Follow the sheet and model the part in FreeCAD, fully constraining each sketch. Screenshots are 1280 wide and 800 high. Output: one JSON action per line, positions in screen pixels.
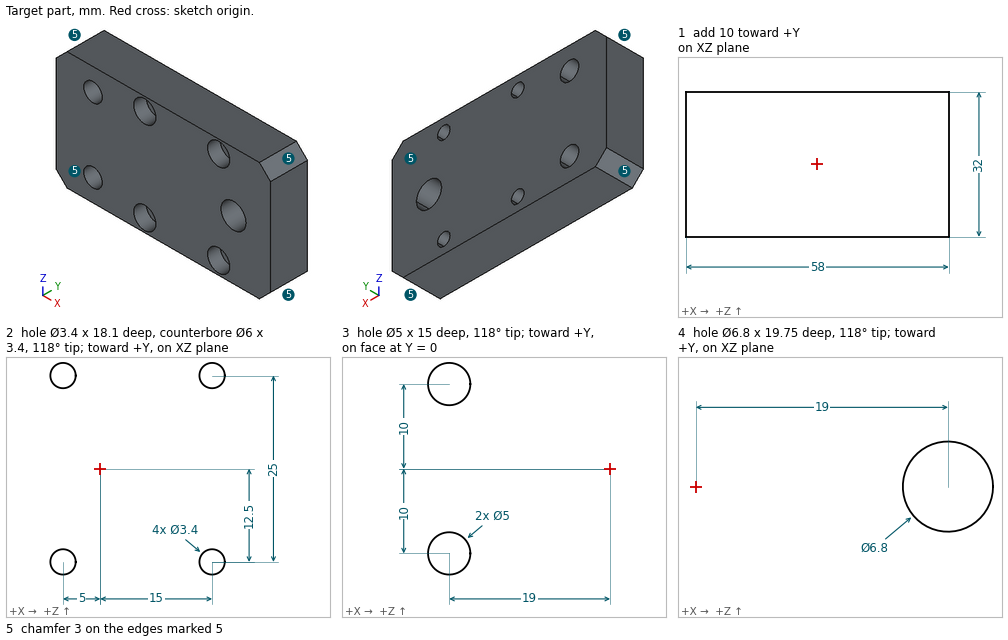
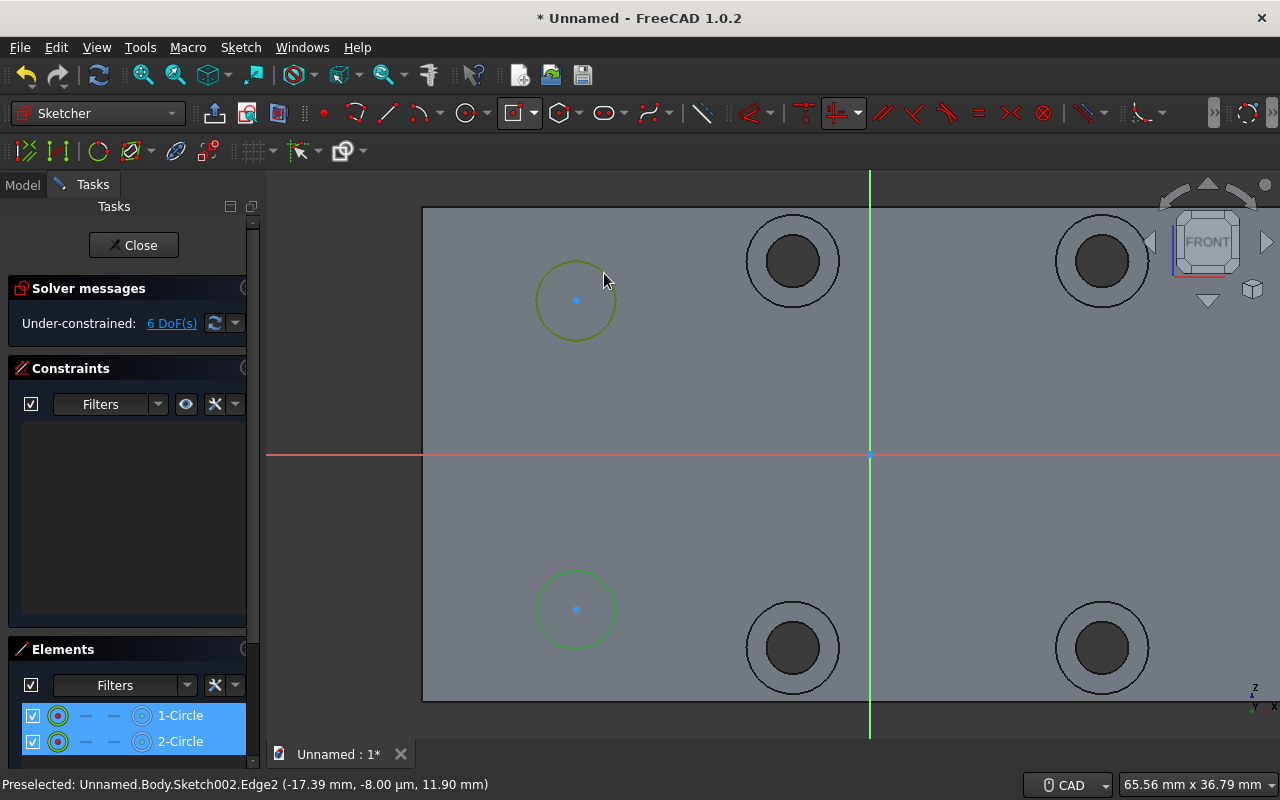
{"action": "left_click", "coordinate": [980, 114]}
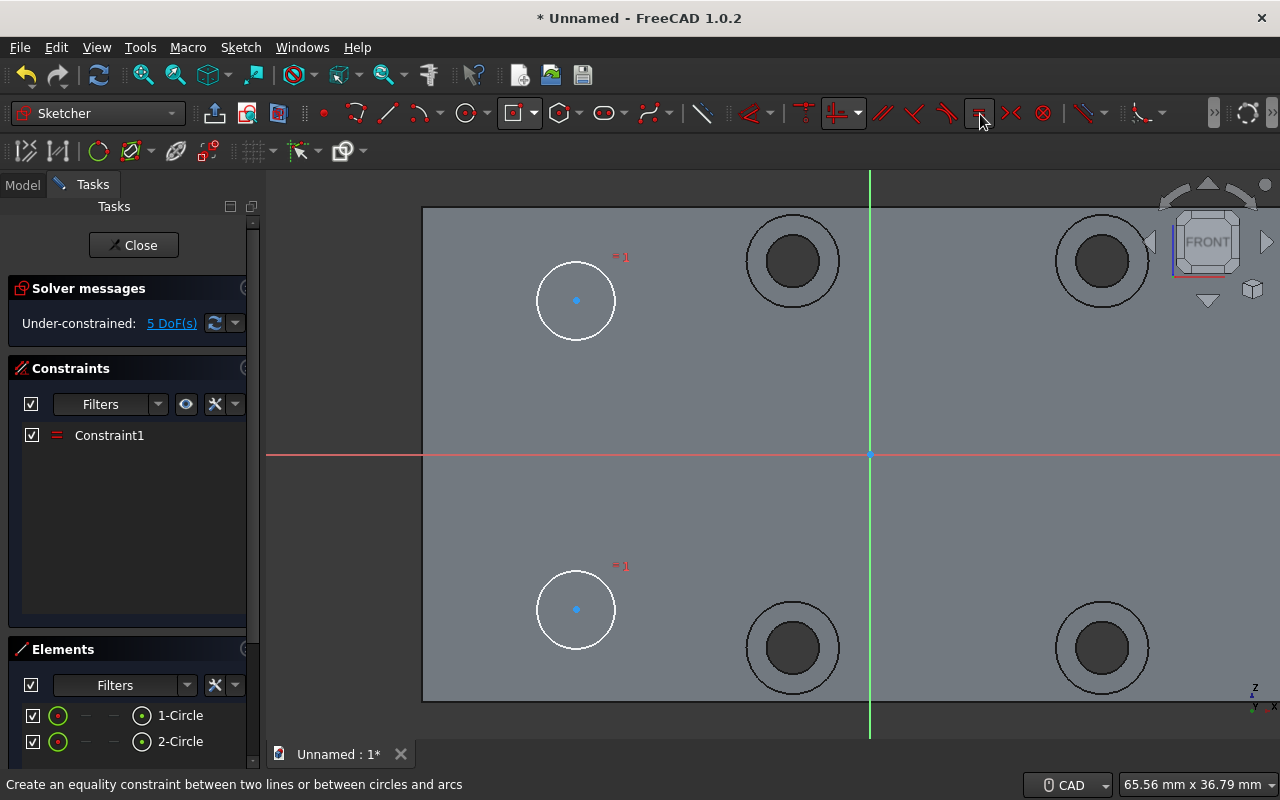
{"action": "left_click", "coordinate": [576, 610]}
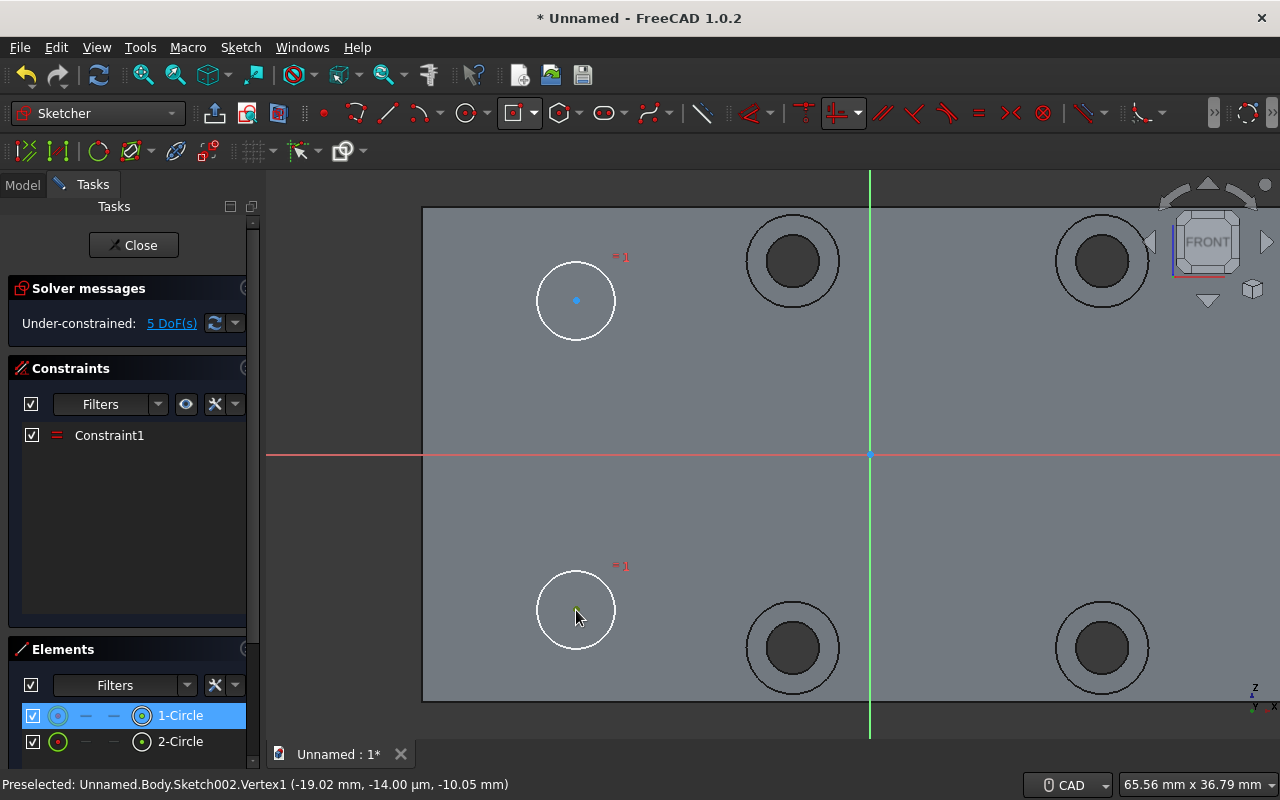
{"action": "left_click", "coordinate": [576, 301]}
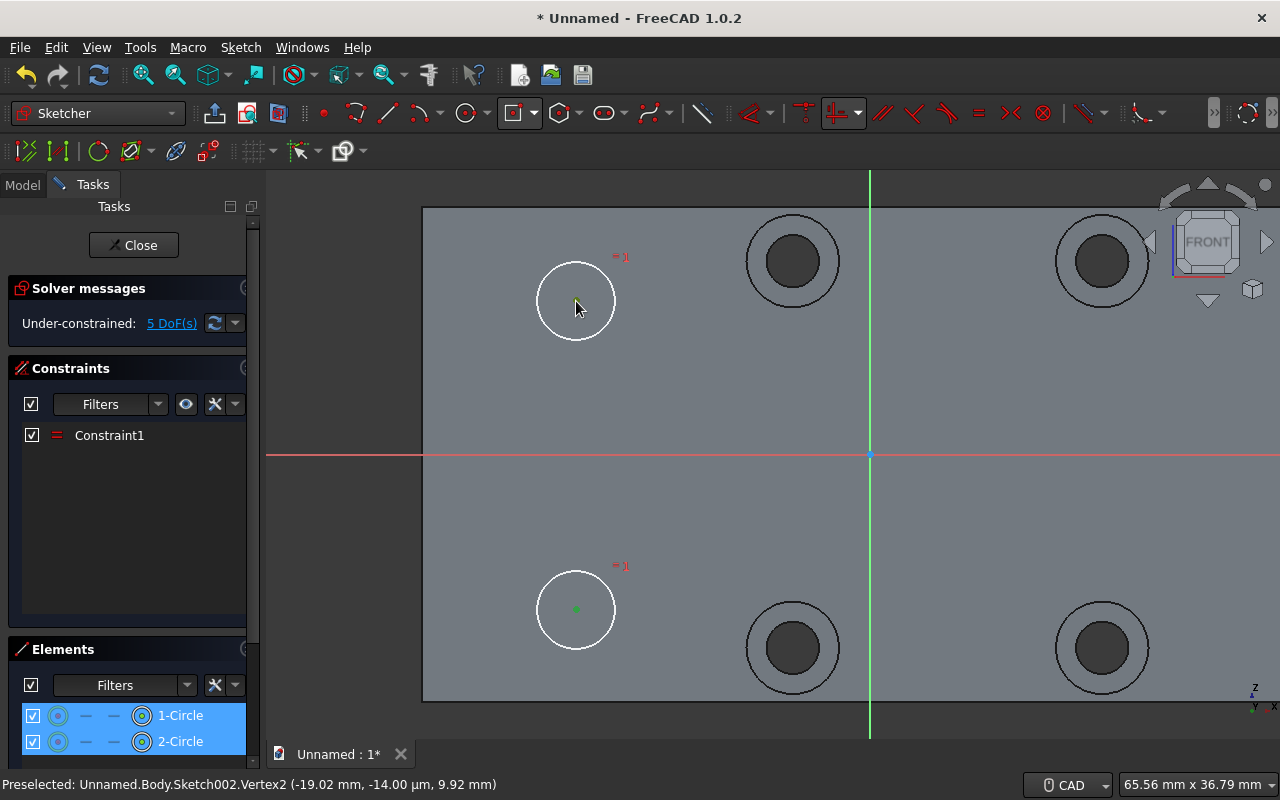
{"action": "key", "text": "v"}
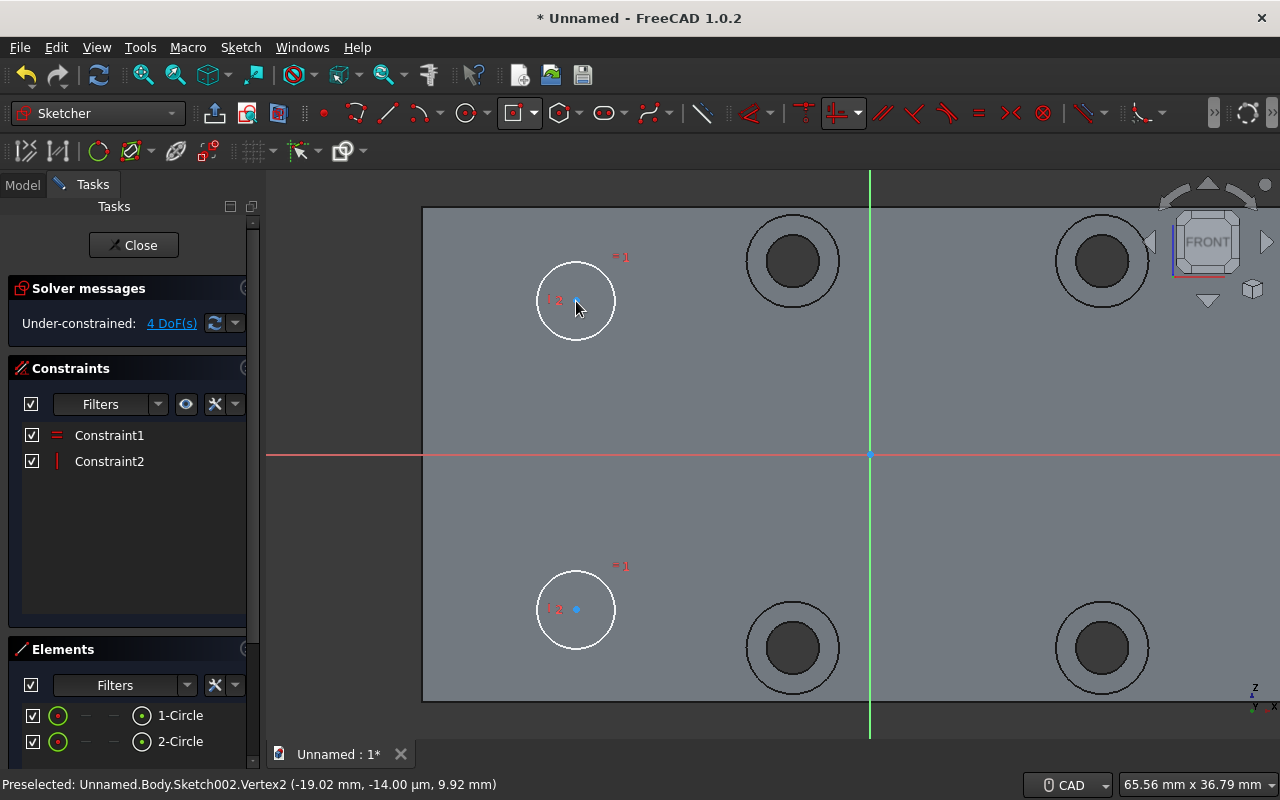
{"action": "left_click", "coordinate": [750, 114]}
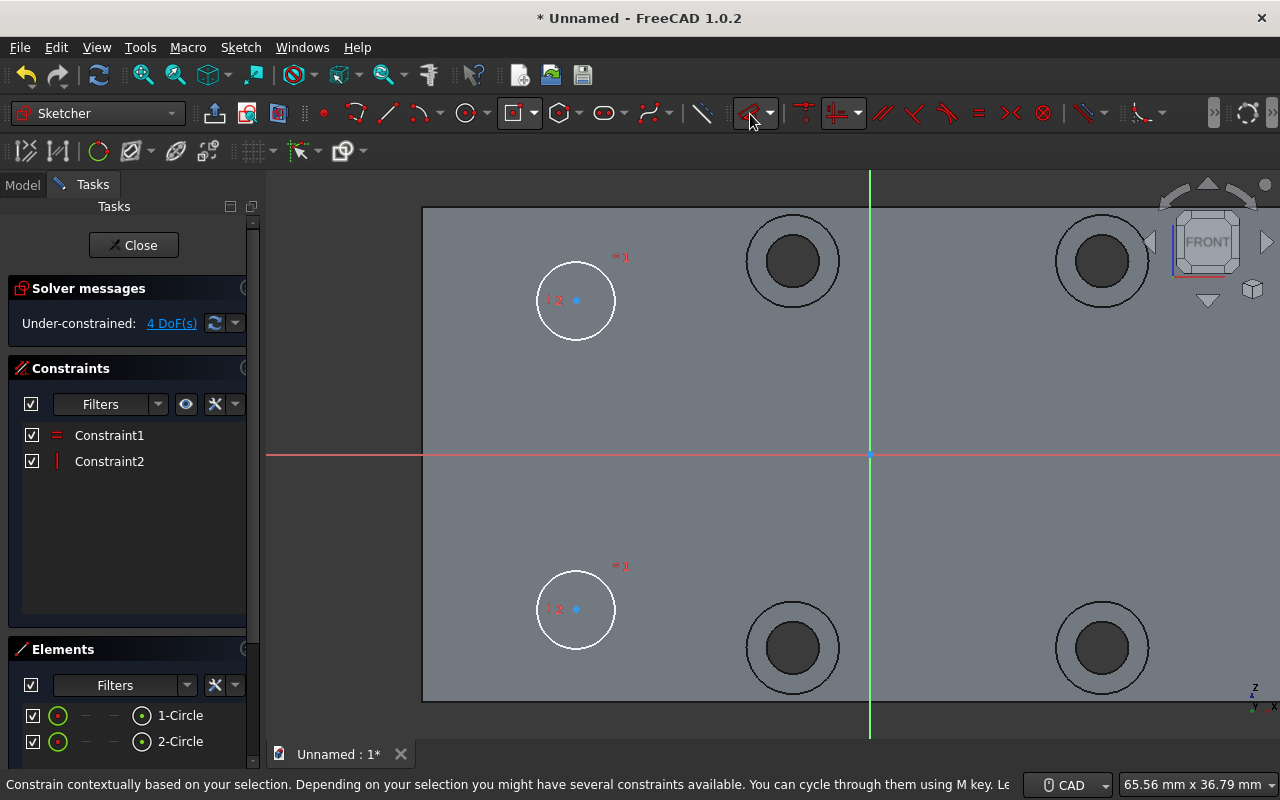
{"action": "left_click", "coordinate": [603, 582]}
{"action": "left_click", "coordinate": [625, 559]}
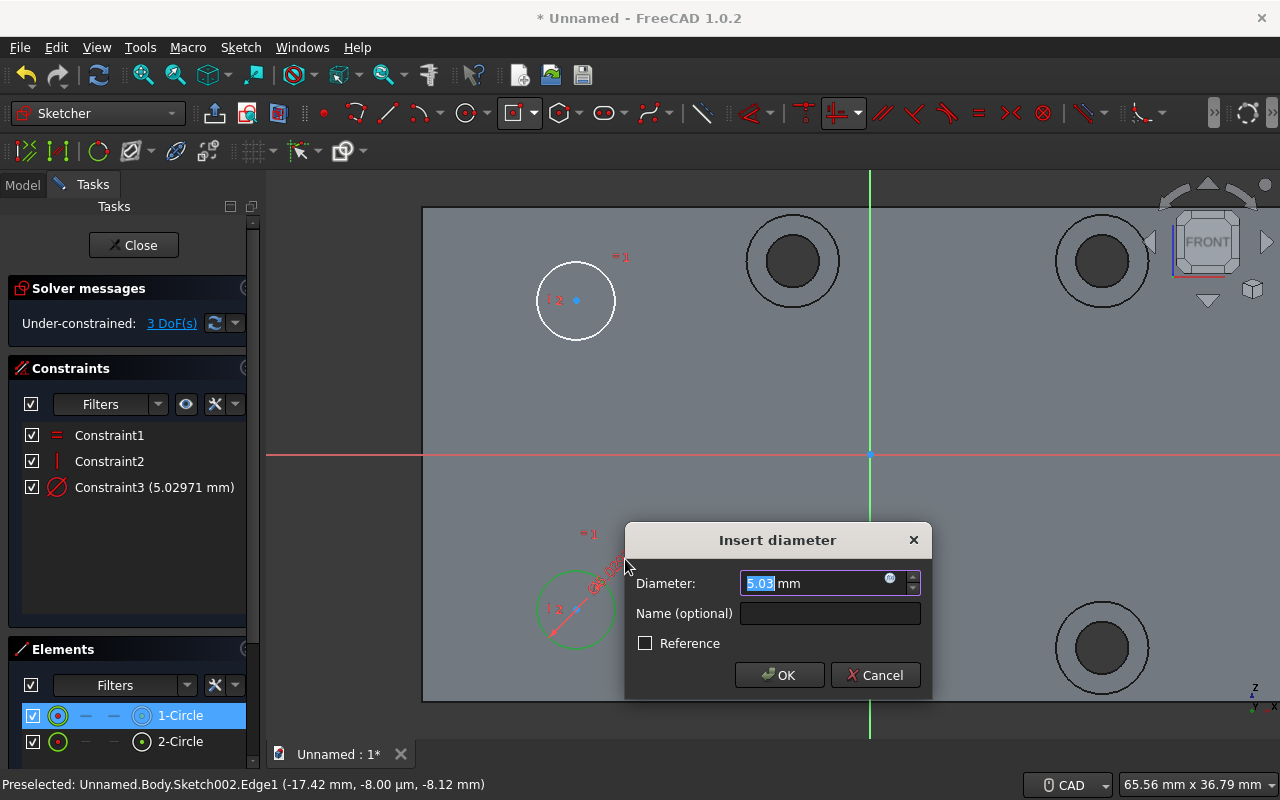
{"action": "type", "text": "5"}
{"action": "key", "text": "Return"}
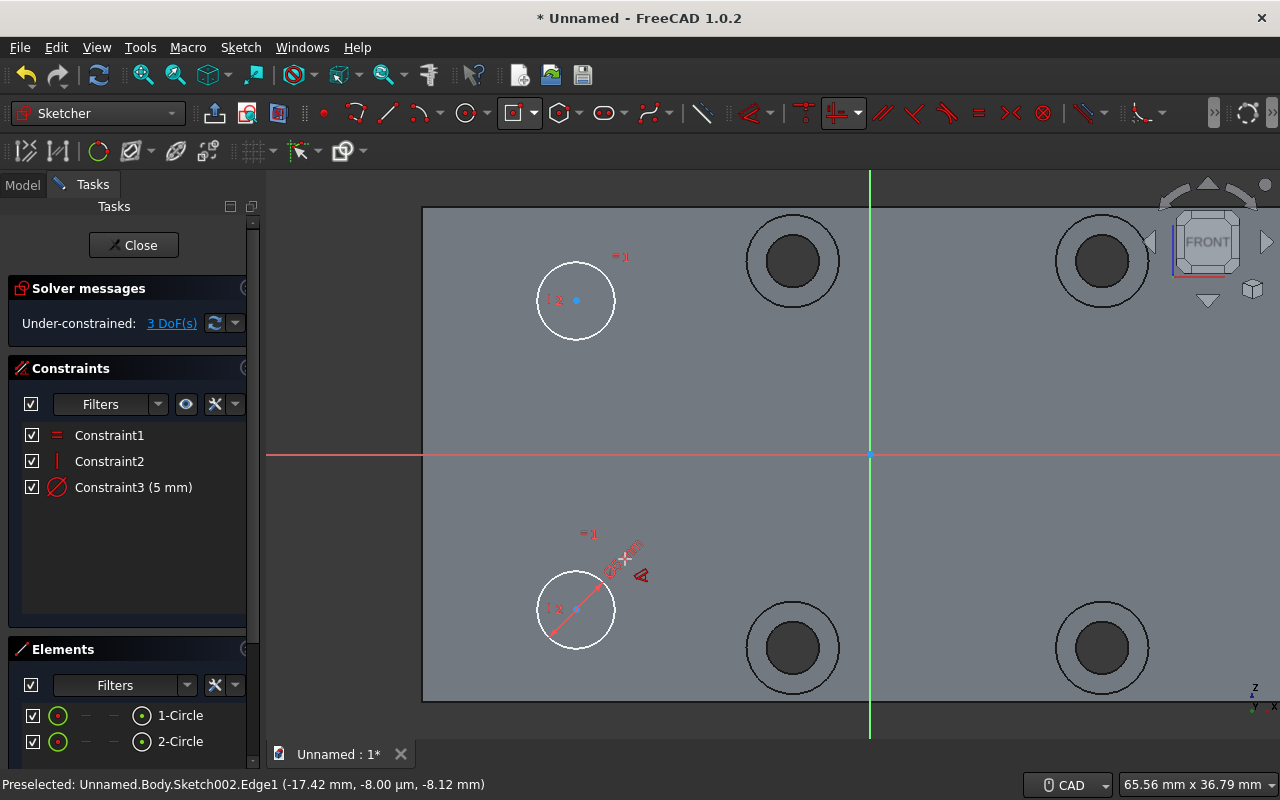
{"action": "left_click", "coordinate": [576, 610]}
{"action": "left_click", "coordinate": [723, 644]}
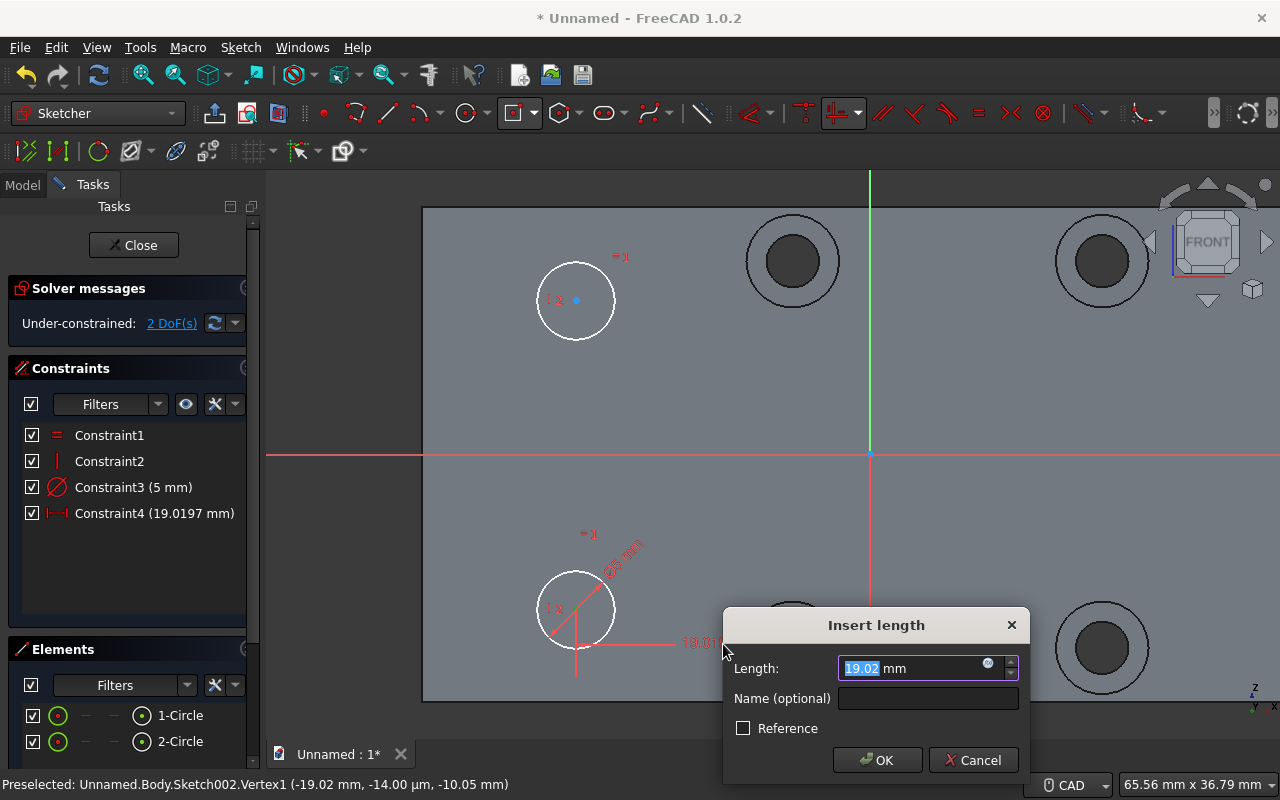
{"action": "type", "text": "19"}
{"action": "key", "text": "Return"}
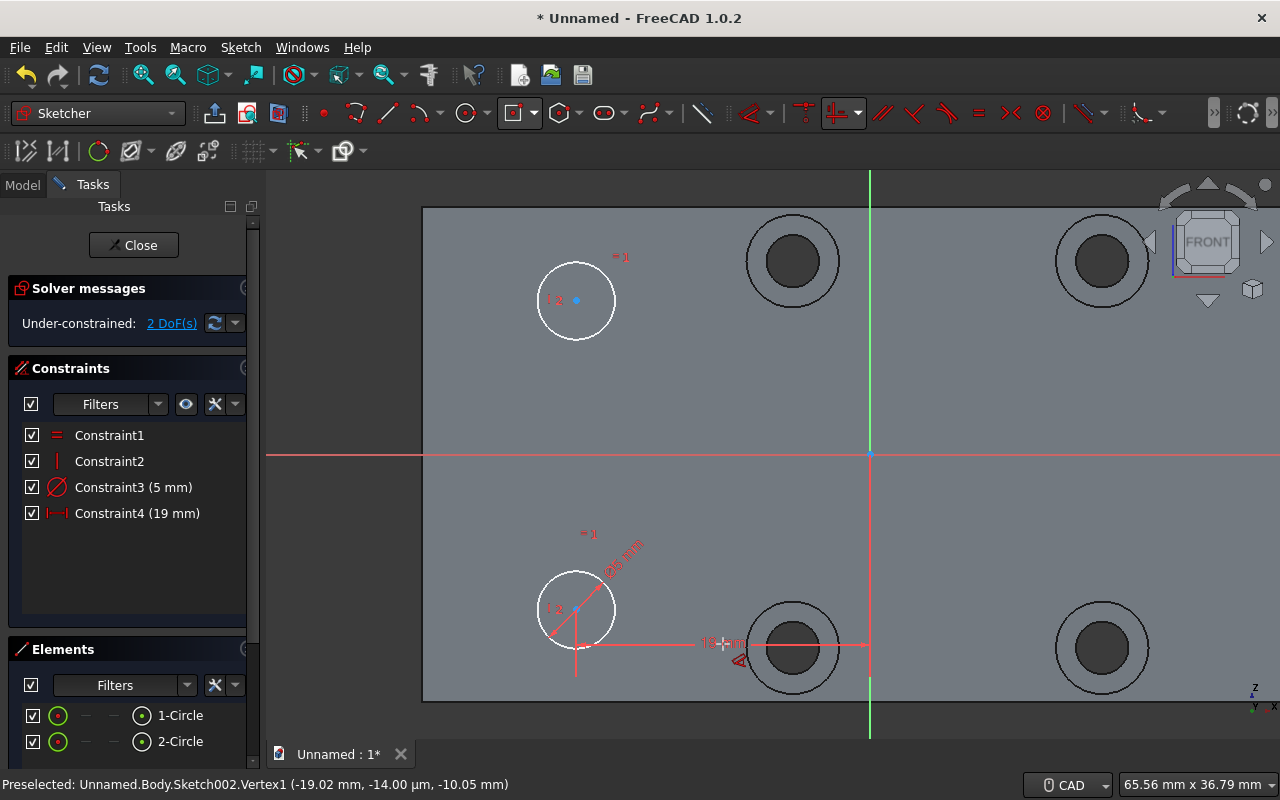
{"action": "left_click", "coordinate": [576, 610]}
{"action": "left_click", "coordinate": [904, 532]}